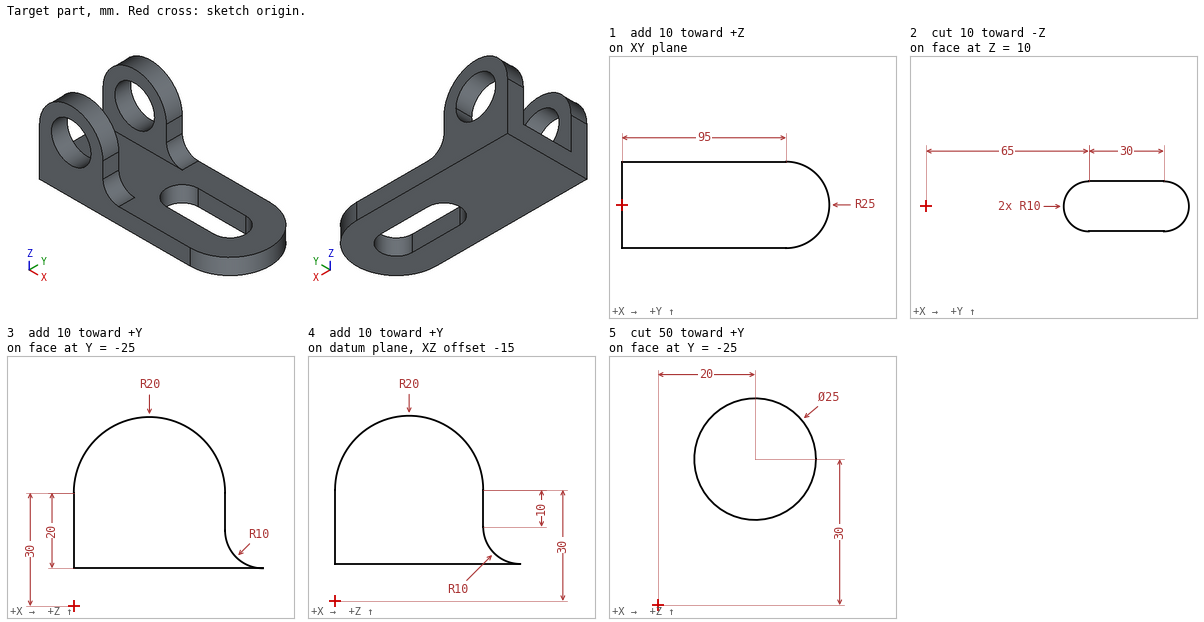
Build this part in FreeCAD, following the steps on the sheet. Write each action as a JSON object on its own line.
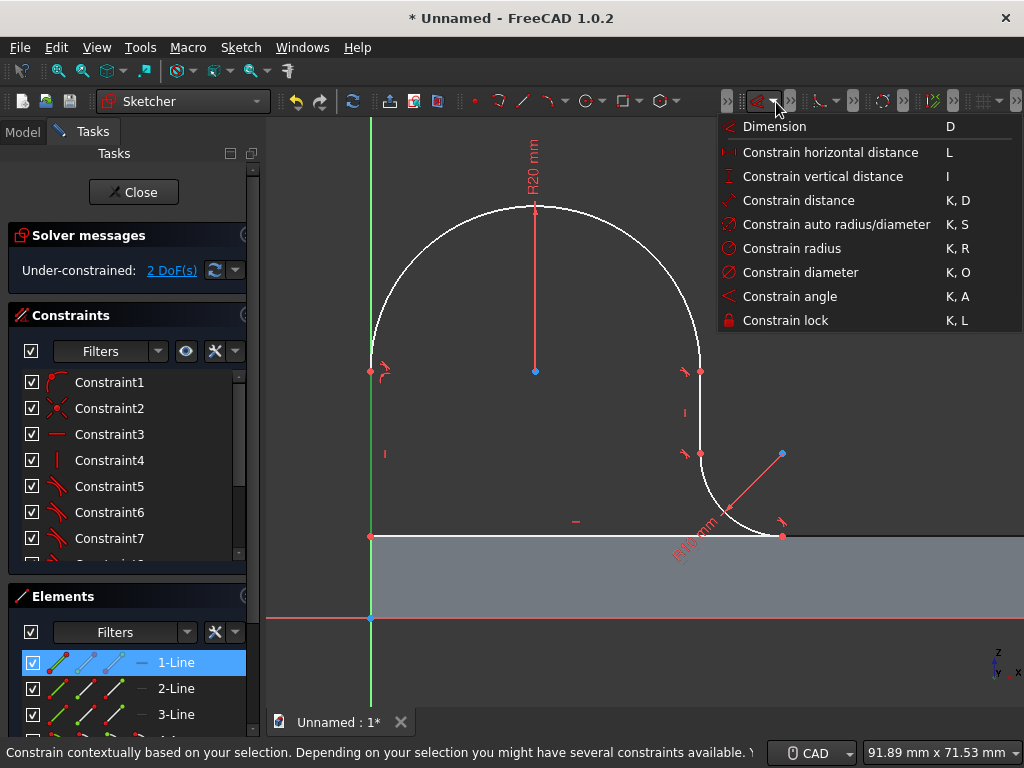
{"action": "left_click", "coordinate": [870, 176]}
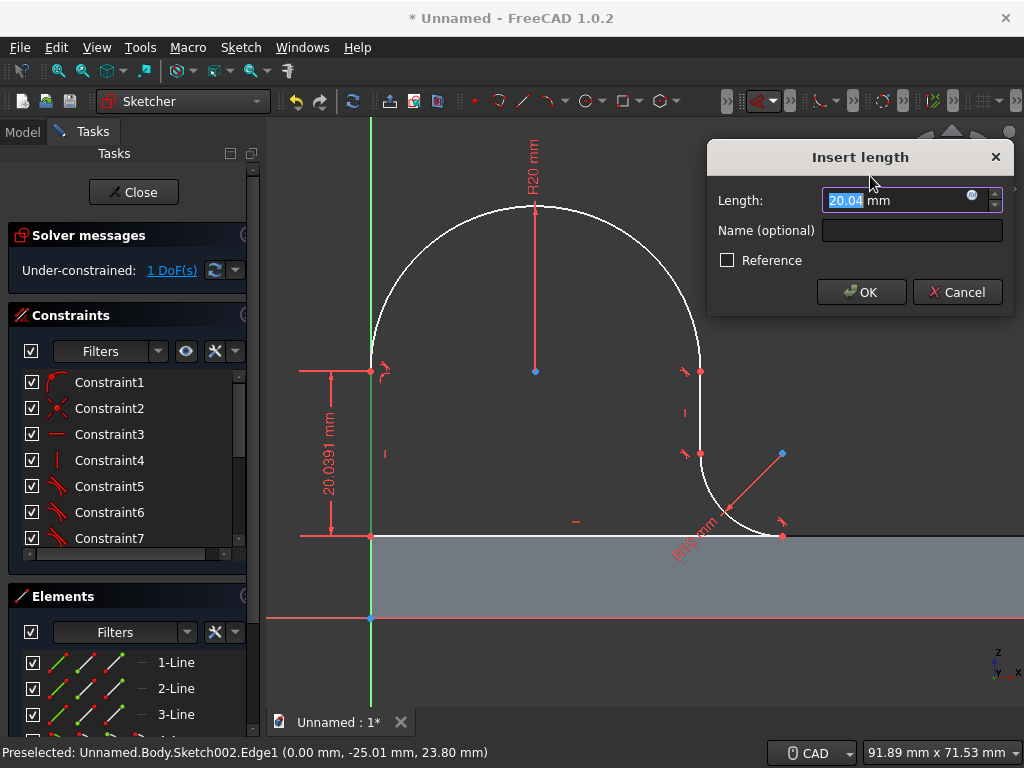
{"action": "type", "text": "20"}
{"action": "key", "text": "Return"}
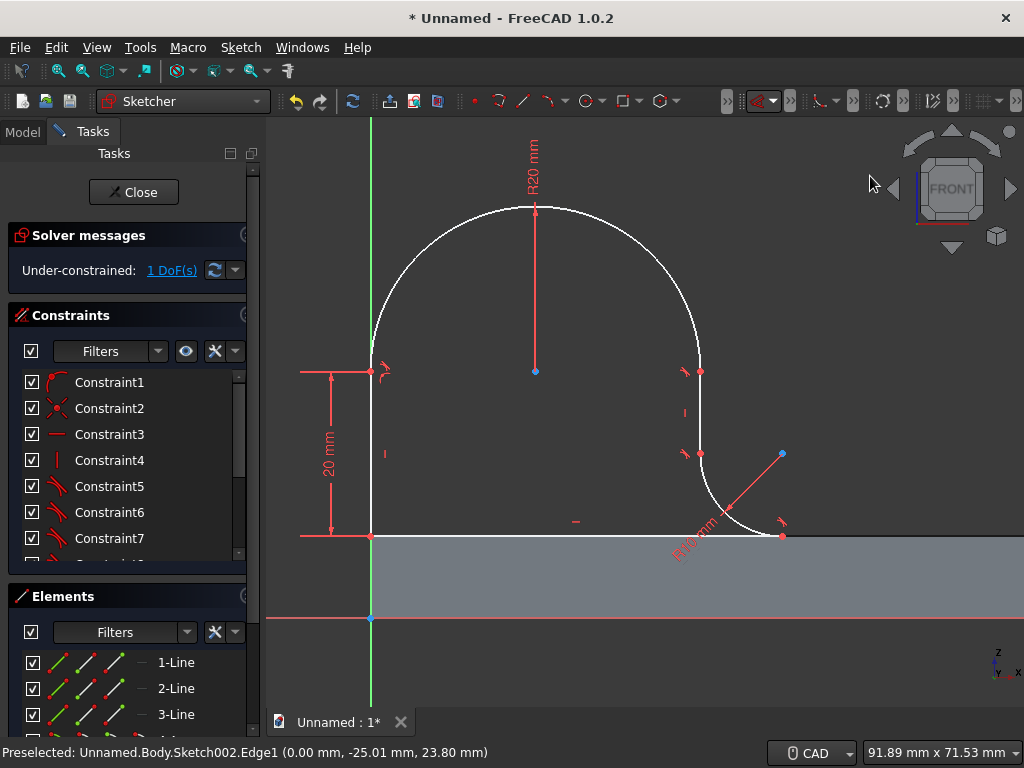
{"action": "left_click", "coordinate": [371, 372]}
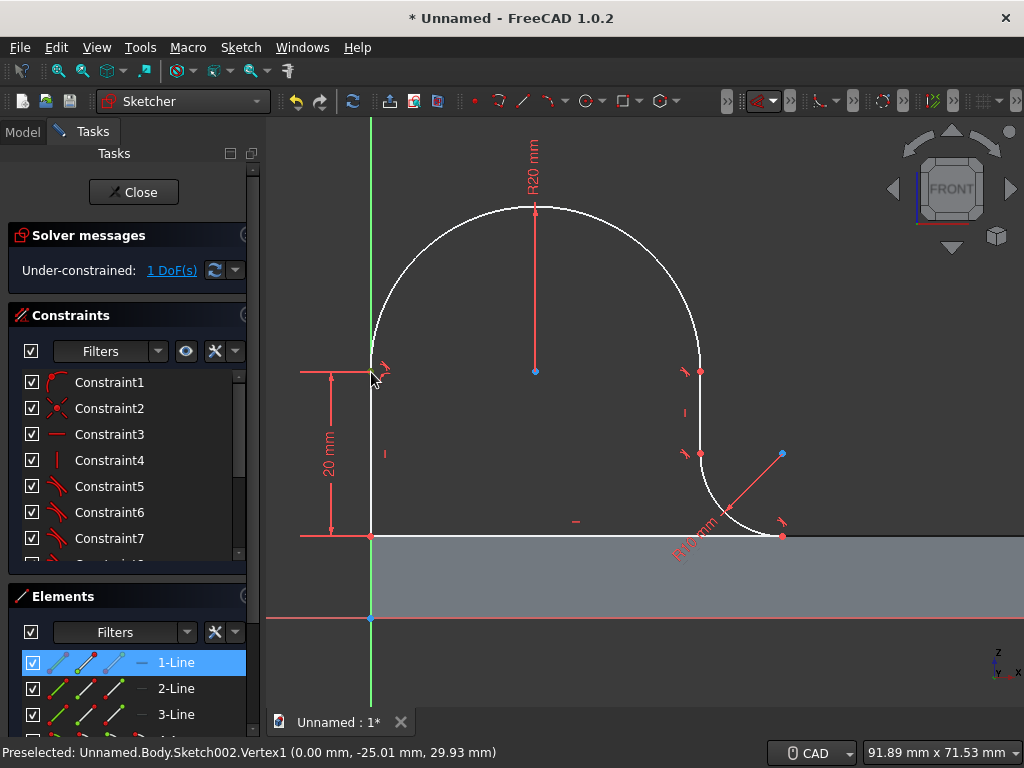
{"action": "key", "text": "i"}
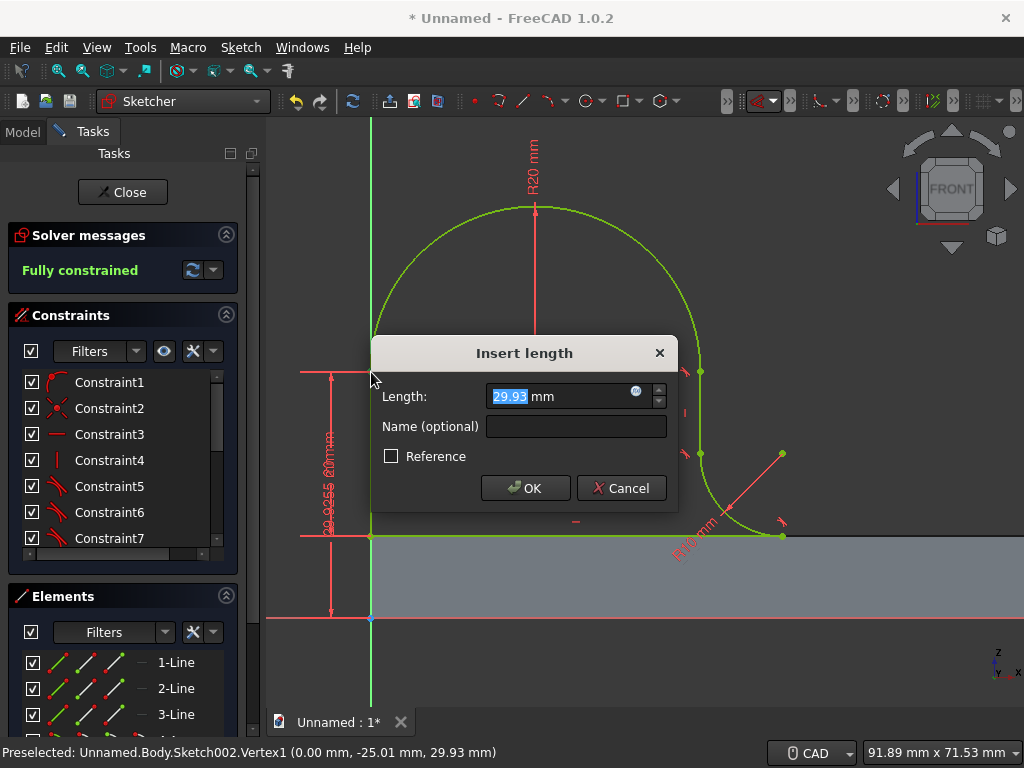
{"action": "type", "text": "30"}
{"action": "key", "text": "Return"}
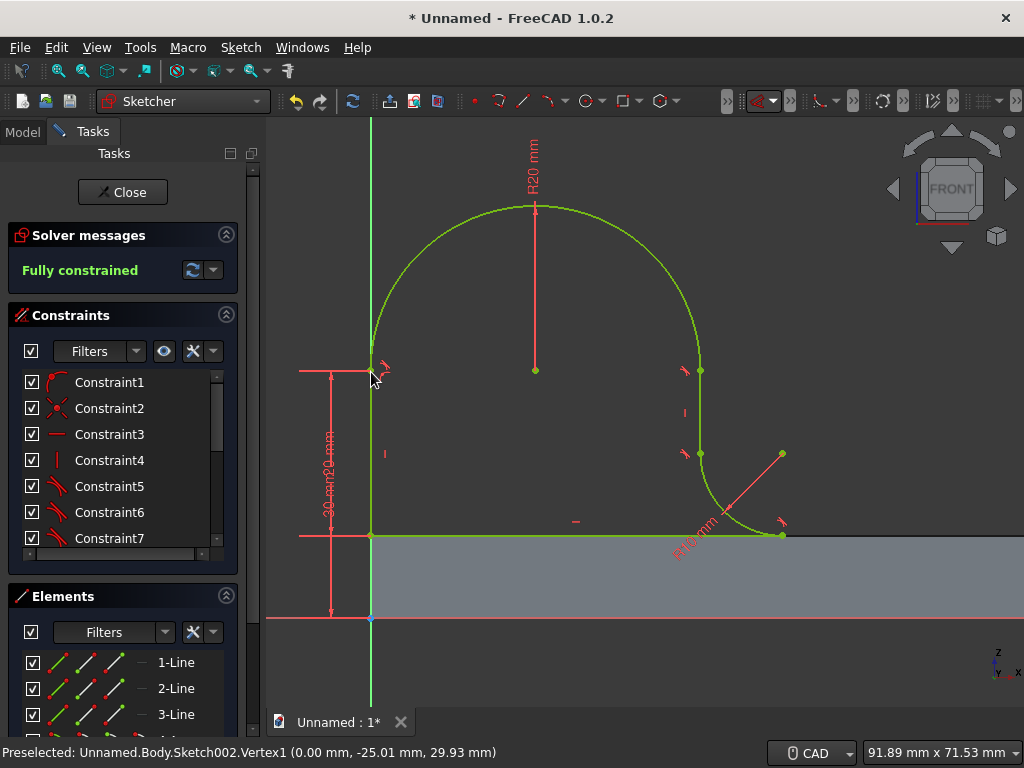
{"action": "left_click", "coordinate": [123, 192]}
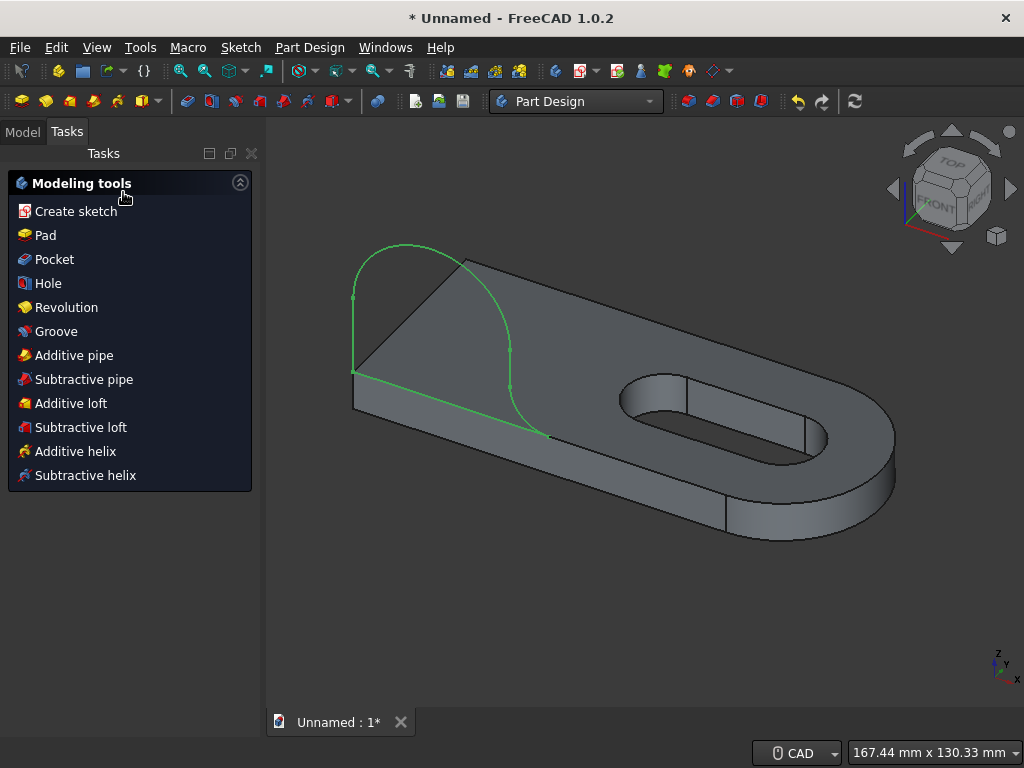
{"action": "left_click", "coordinate": [22, 102]}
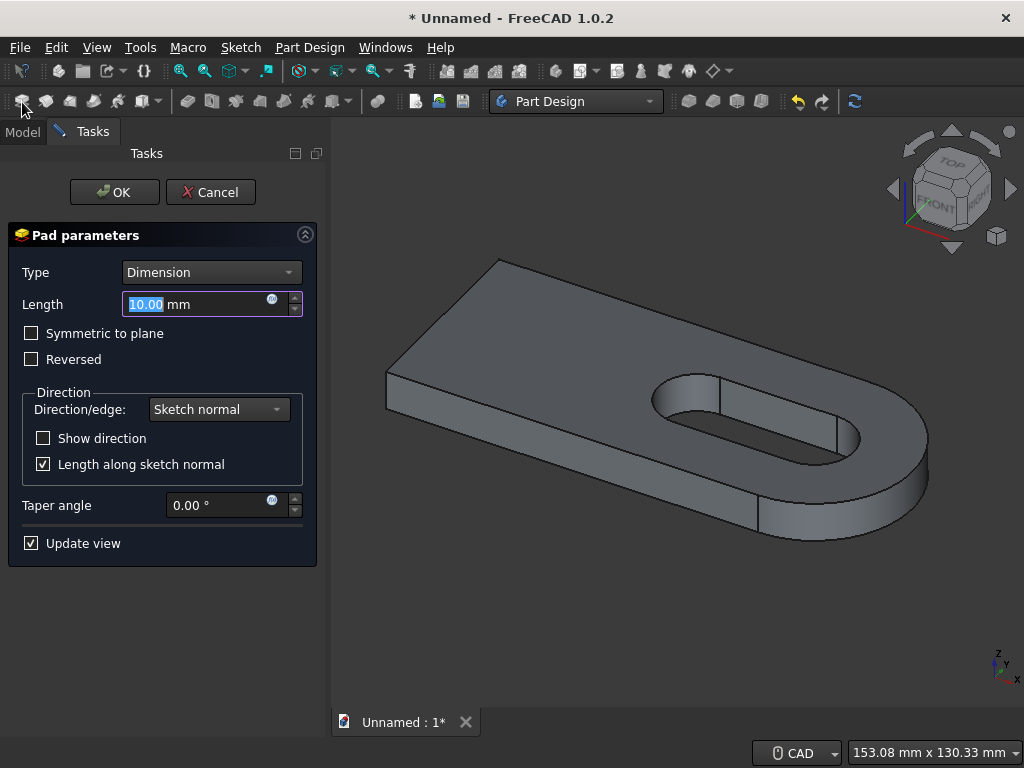
{"action": "type", "text": "10"}
{"action": "key", "text": "Tab"}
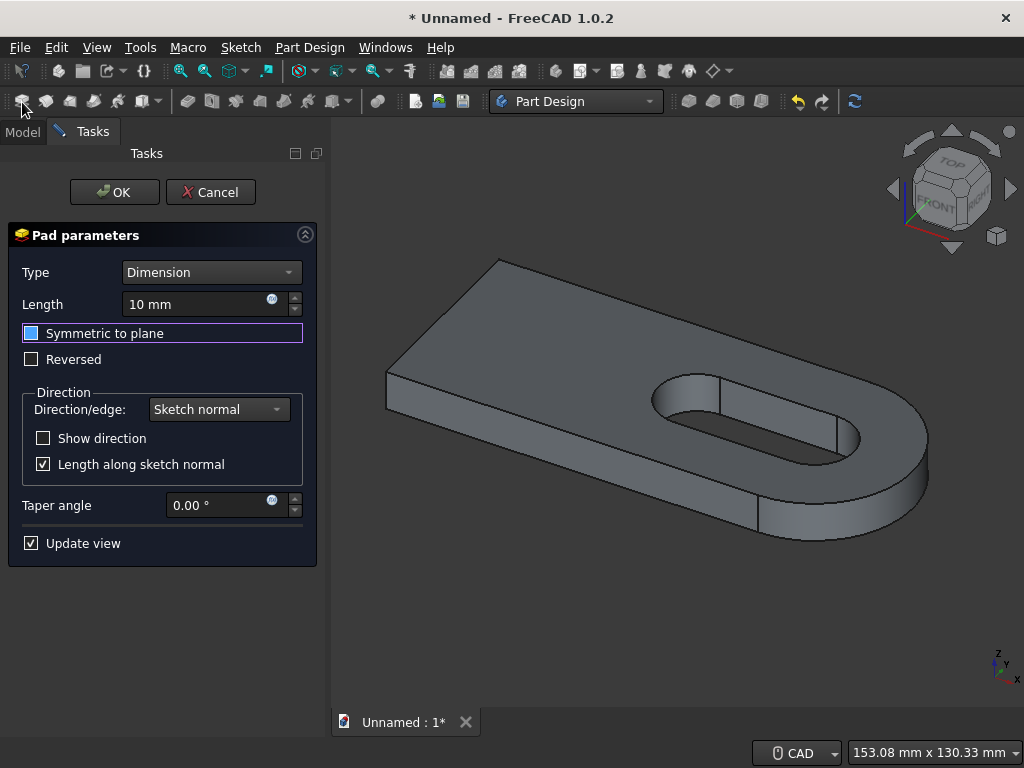
{"action": "left_click", "coordinate": [30, 359]}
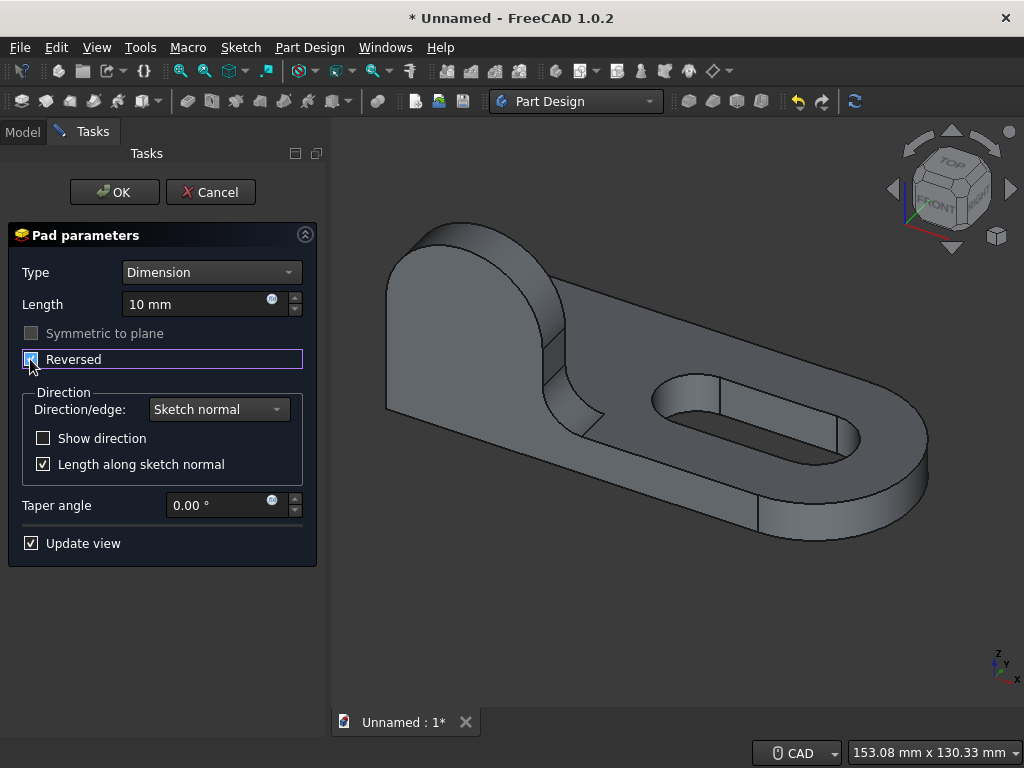
{"action": "left_click", "coordinate": [115, 192]}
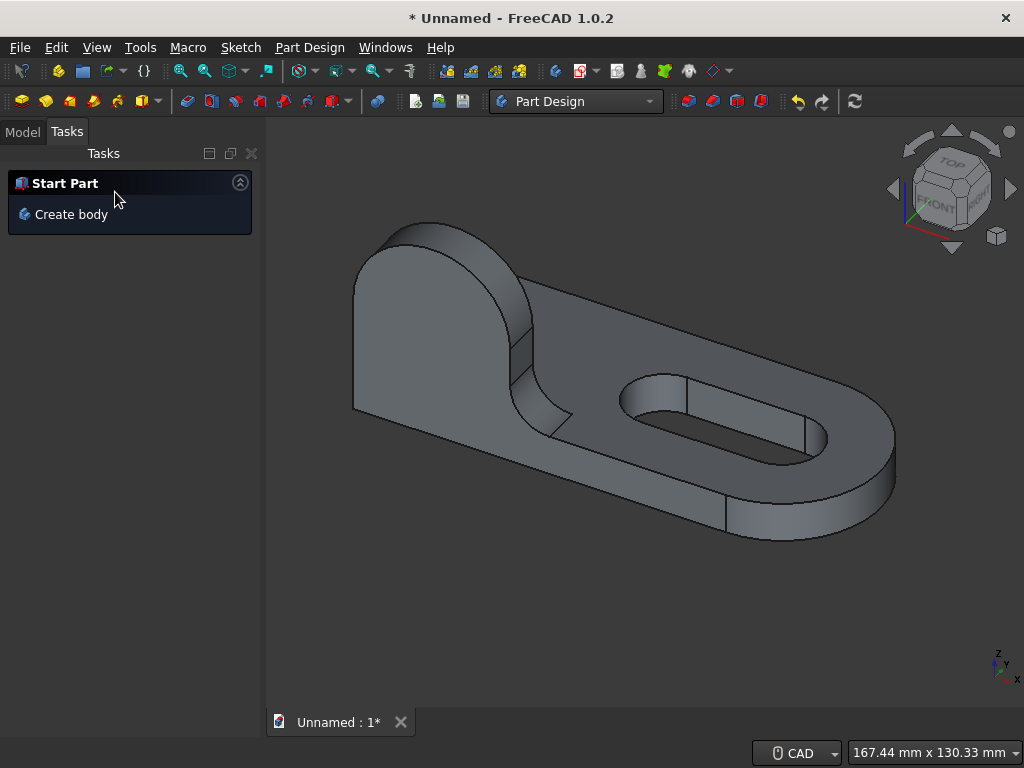
{"action": "left_click", "coordinate": [182, 72]}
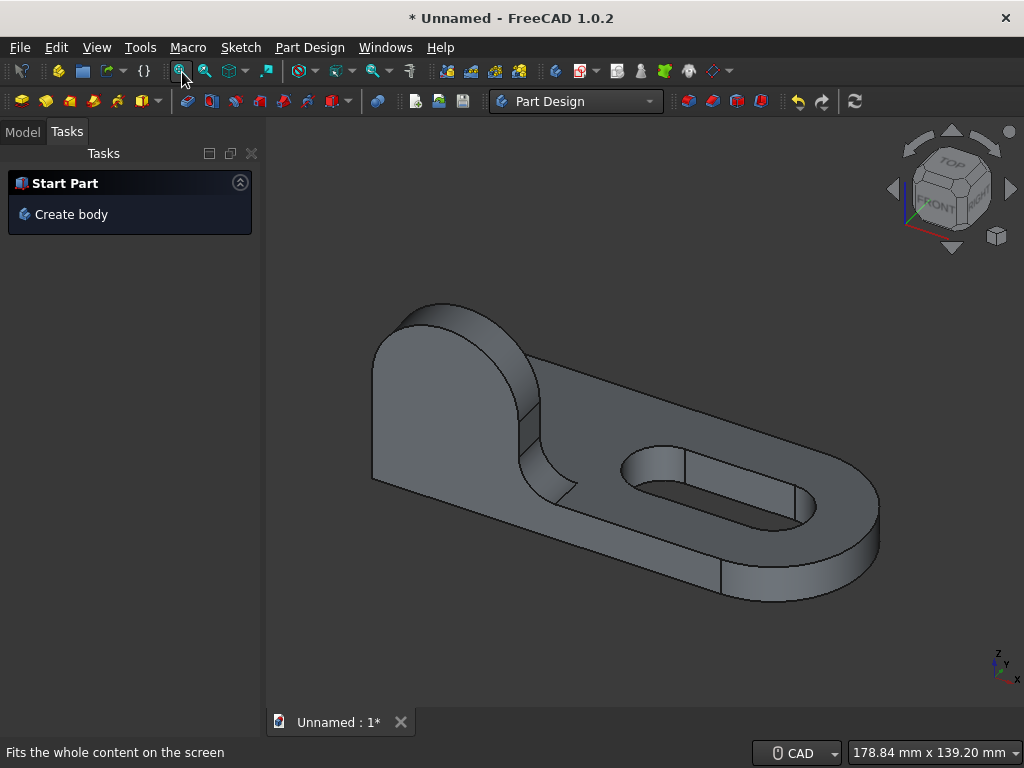
{"action": "left_click", "coordinate": [23, 131]}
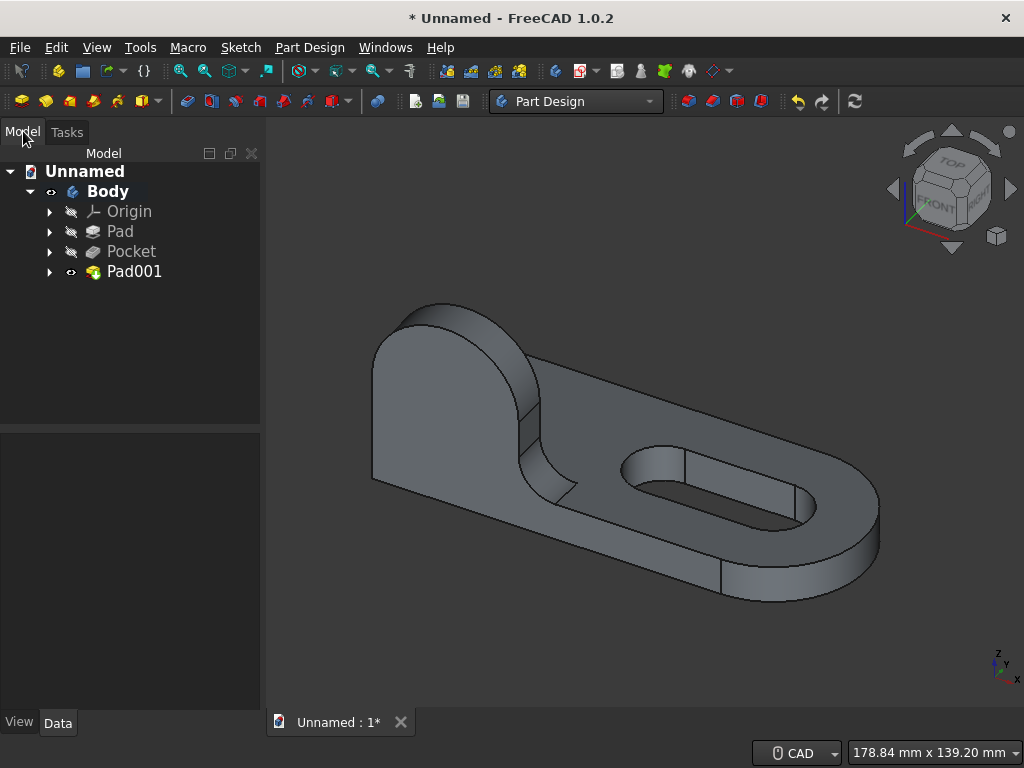
{"action": "left_click", "coordinate": [50, 212]}